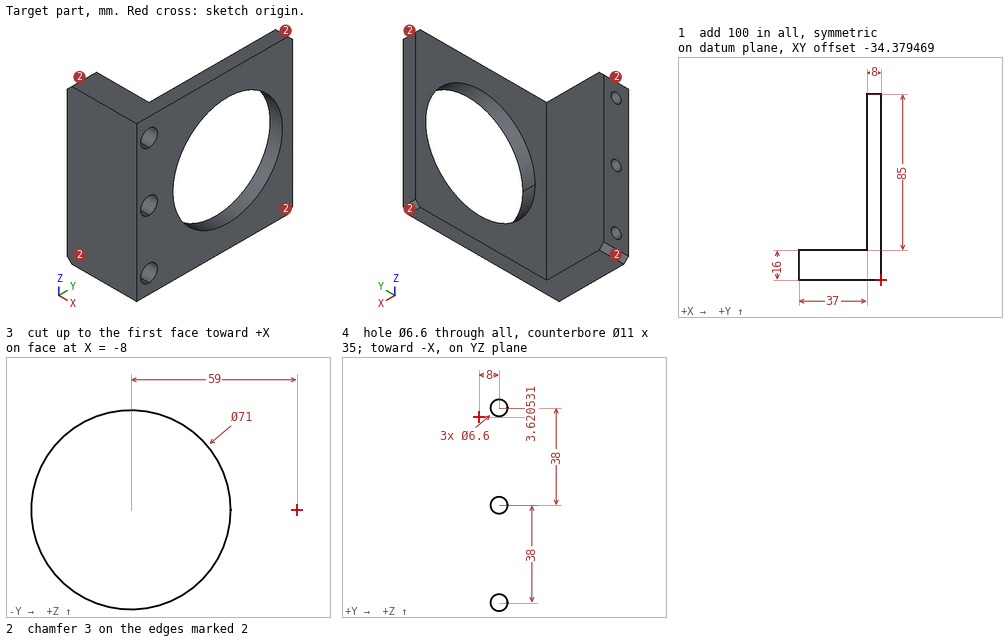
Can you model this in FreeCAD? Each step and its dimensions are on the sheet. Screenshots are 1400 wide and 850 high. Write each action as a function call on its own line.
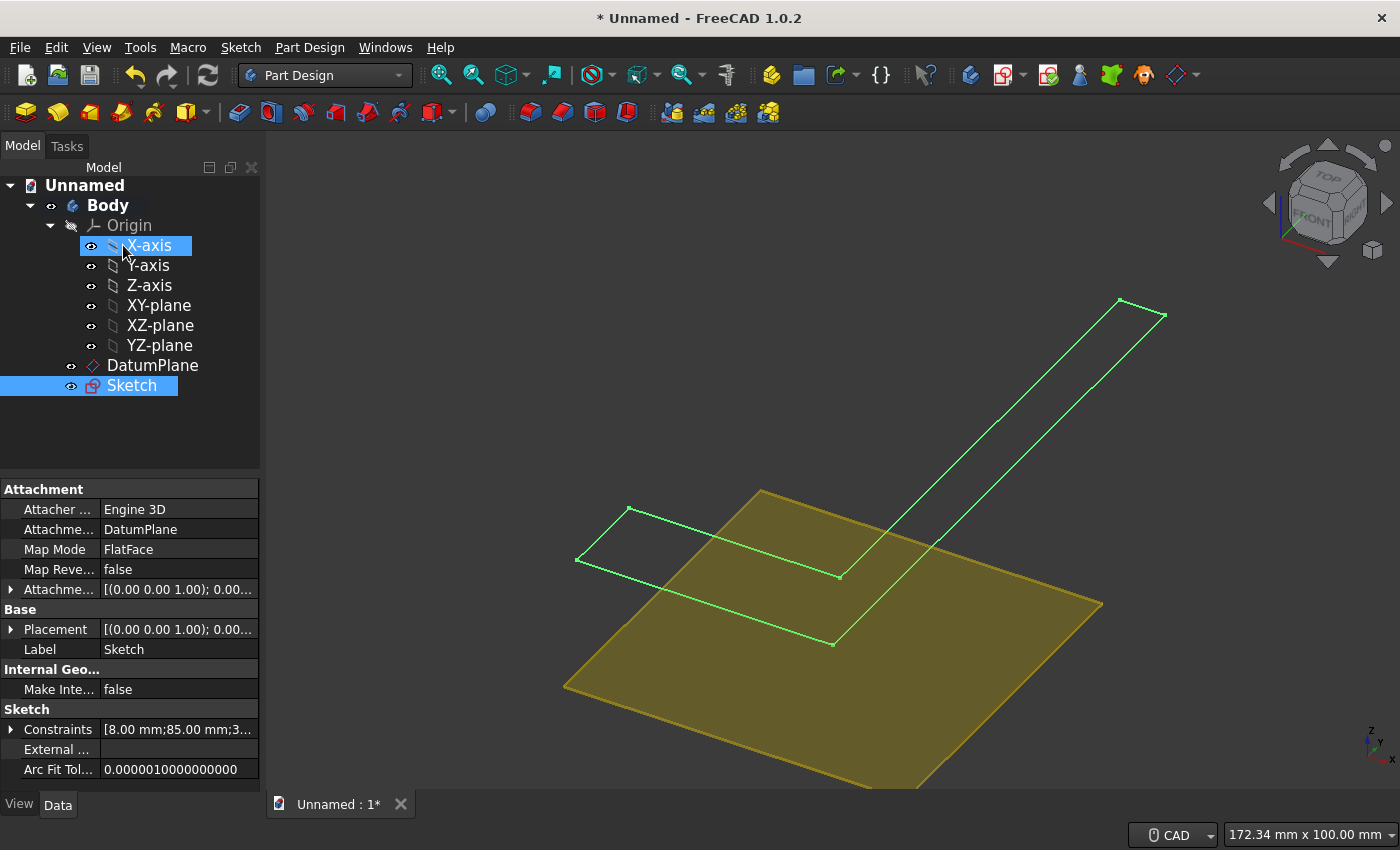
click(26, 112)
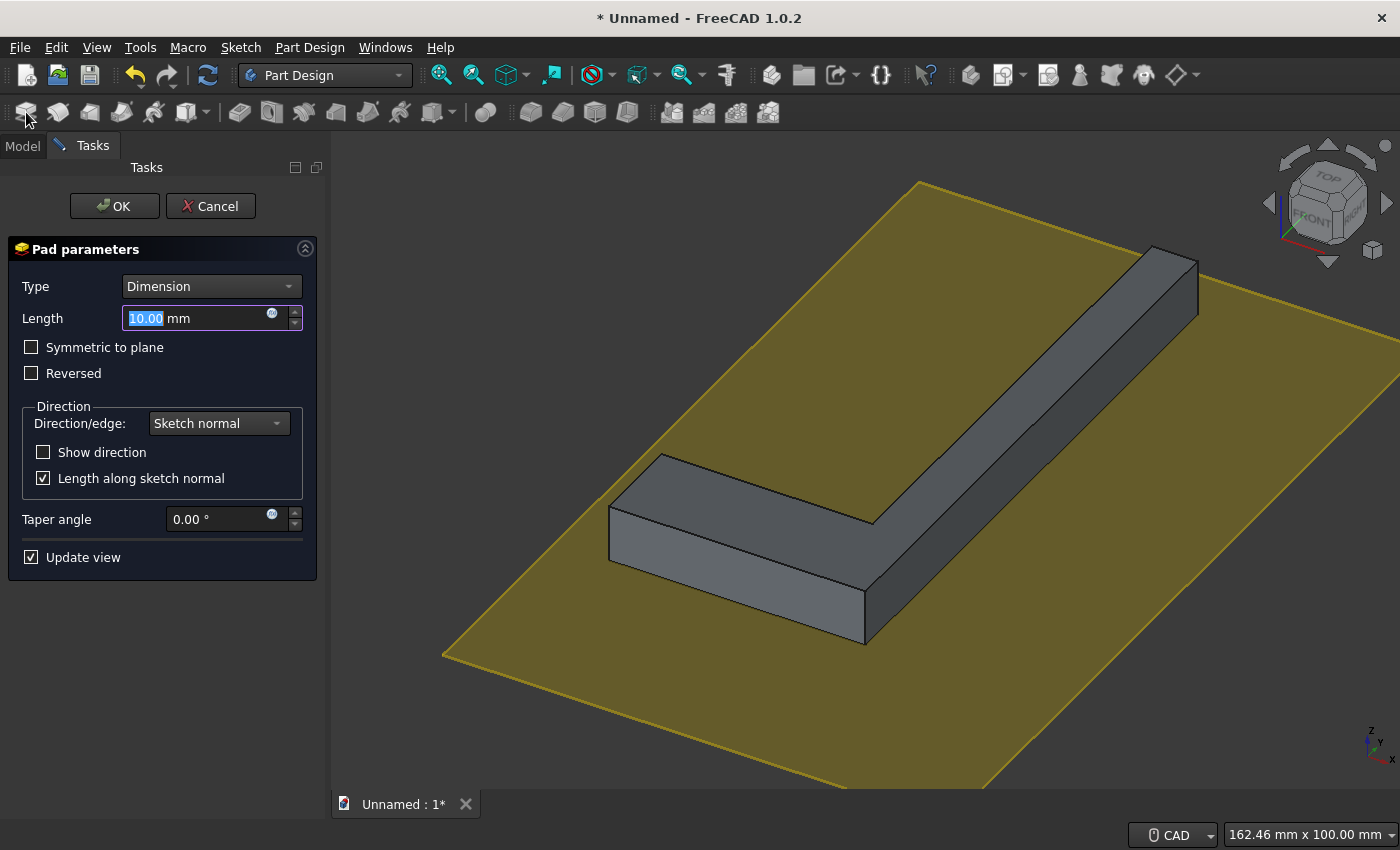
text(100)
key(Tab)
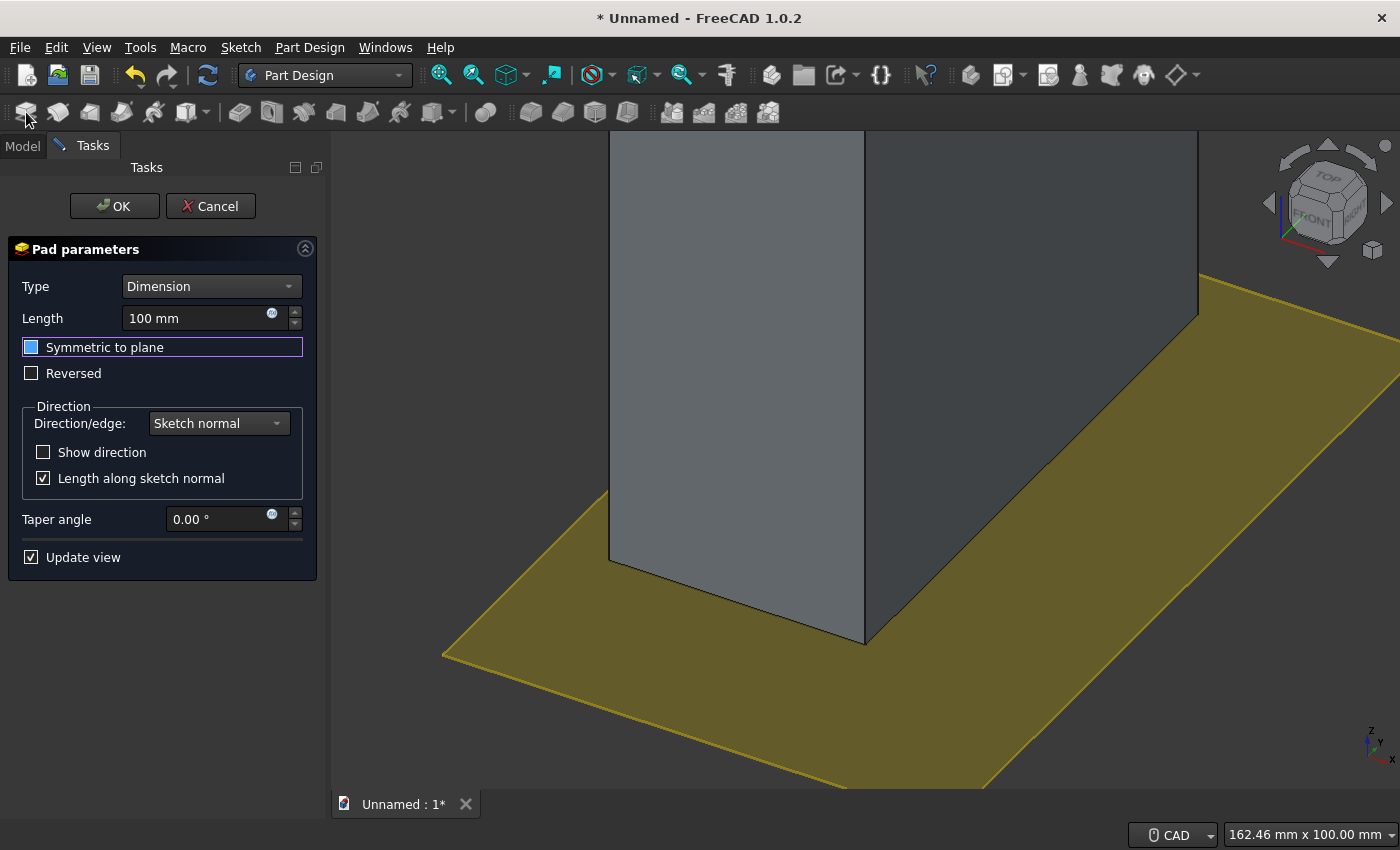
click(30, 347)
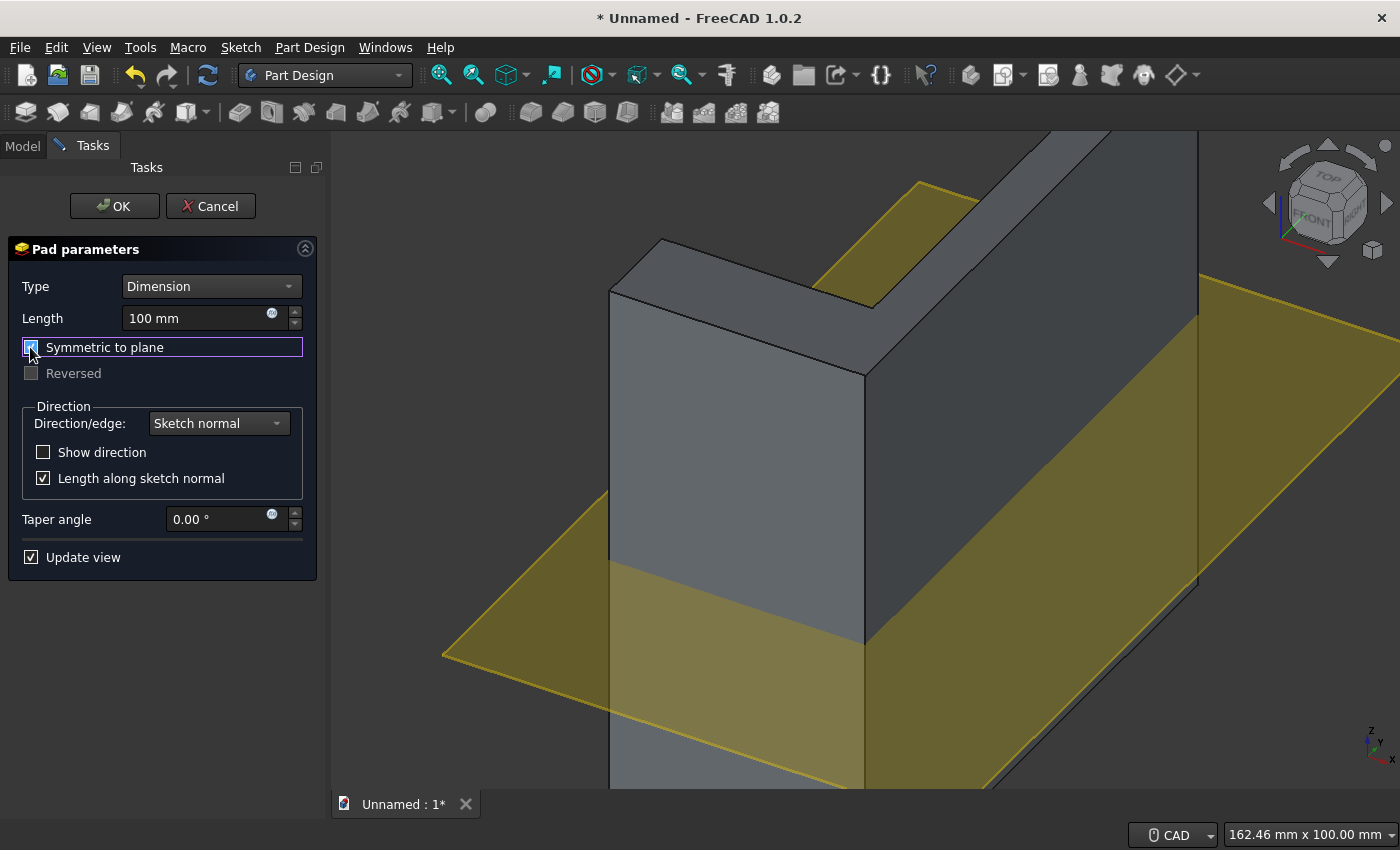
click(115, 206)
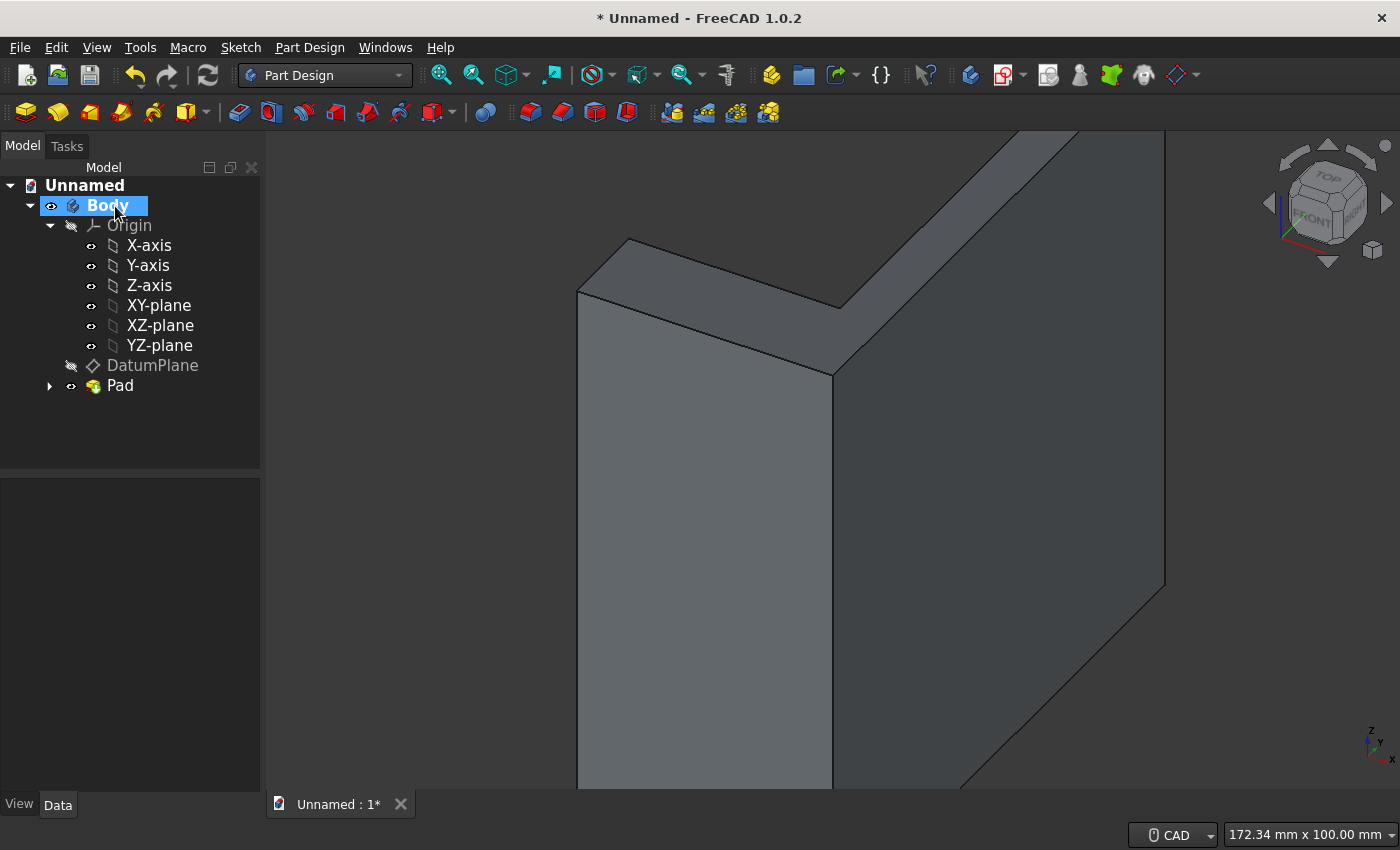
click(442, 76)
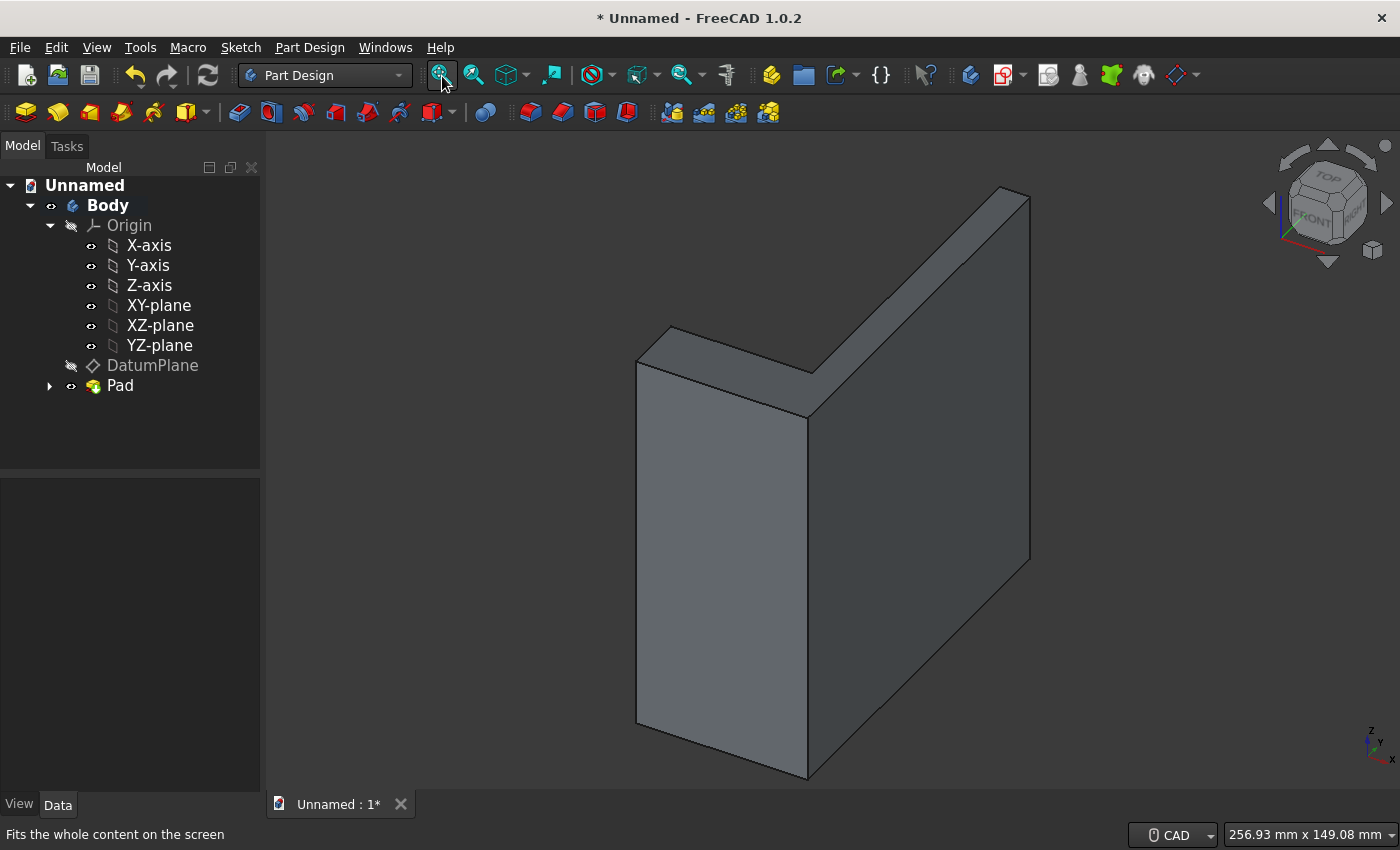
key(0)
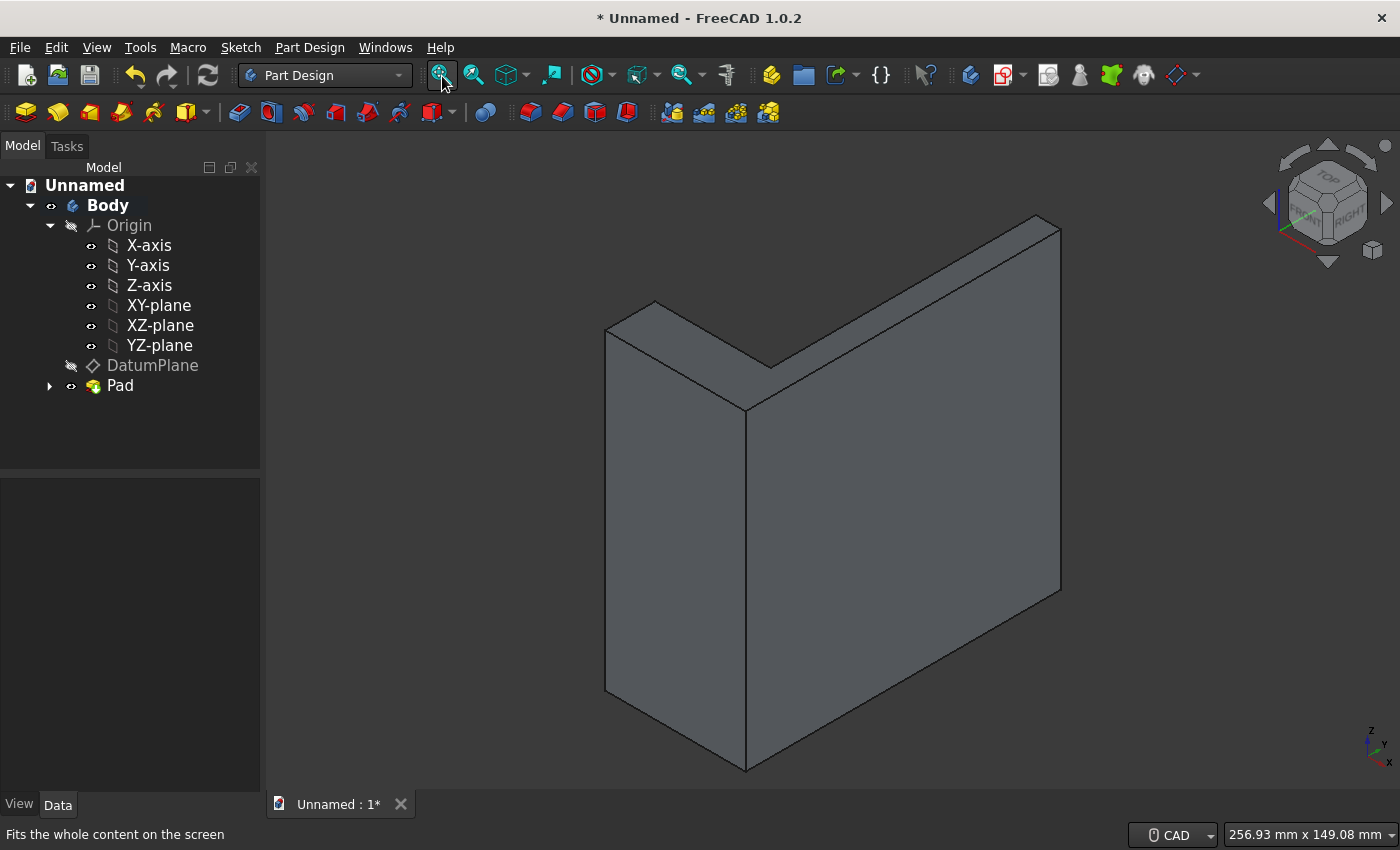
key(2)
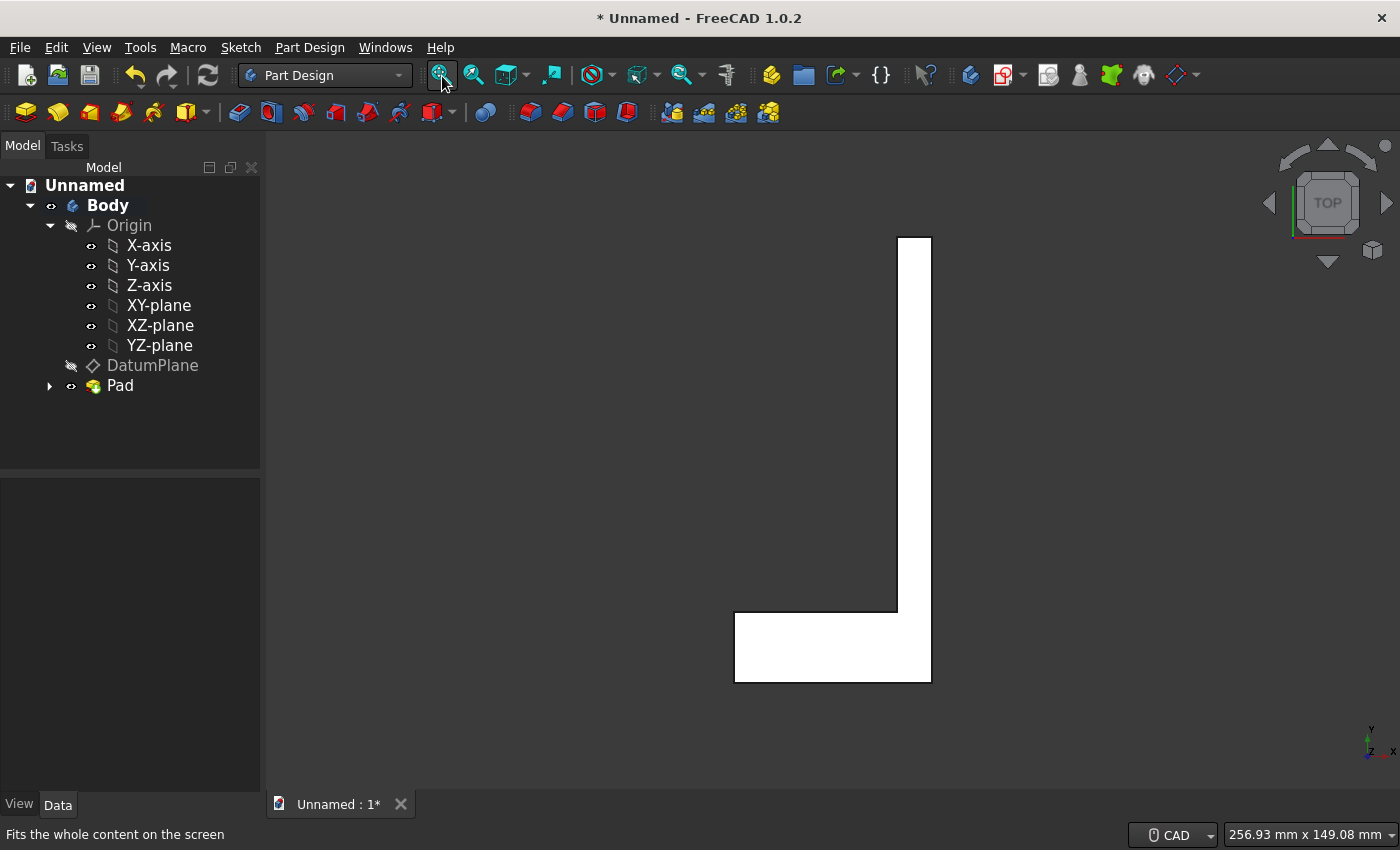
click(734, 647)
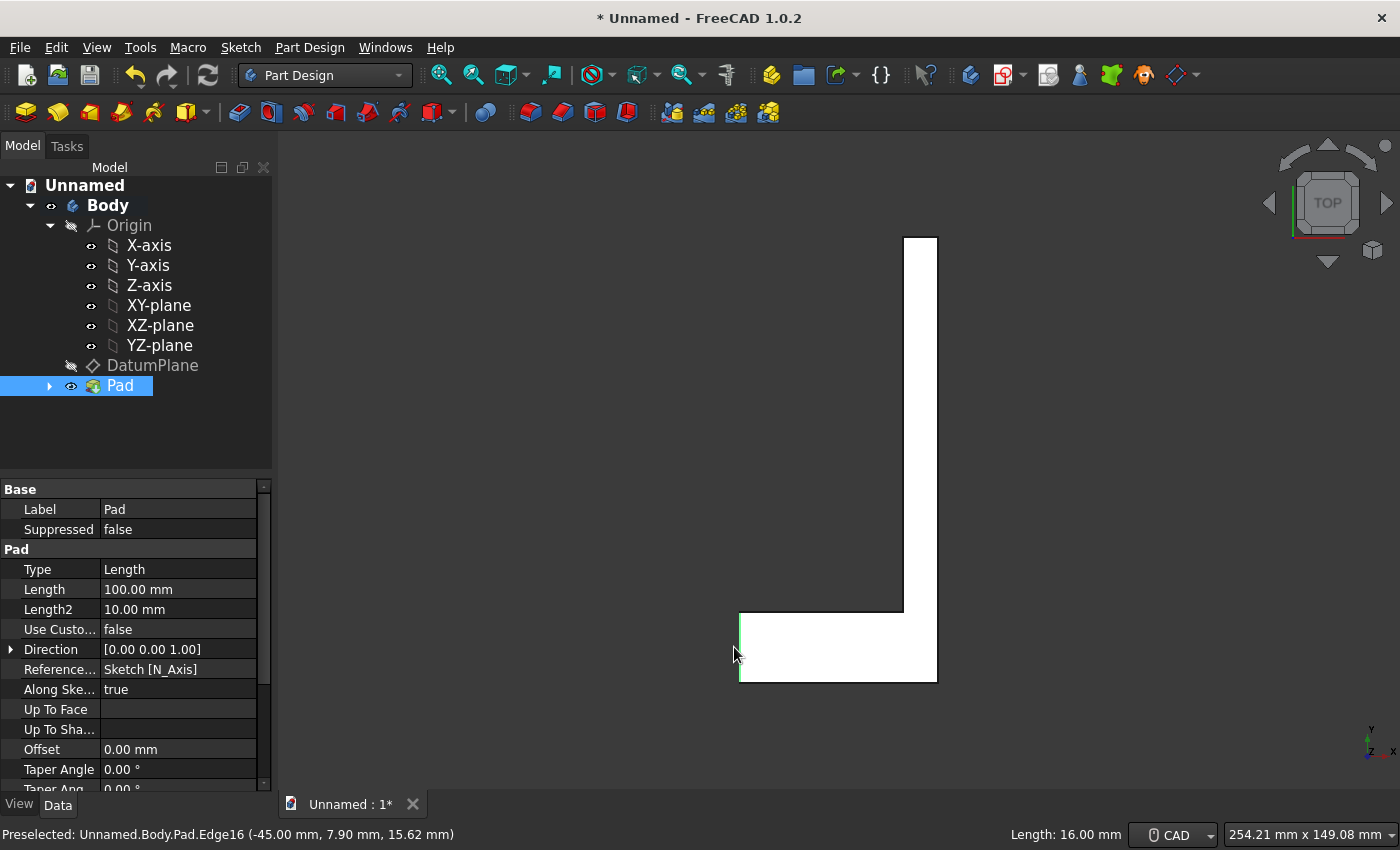
click(921, 236, ctrl)